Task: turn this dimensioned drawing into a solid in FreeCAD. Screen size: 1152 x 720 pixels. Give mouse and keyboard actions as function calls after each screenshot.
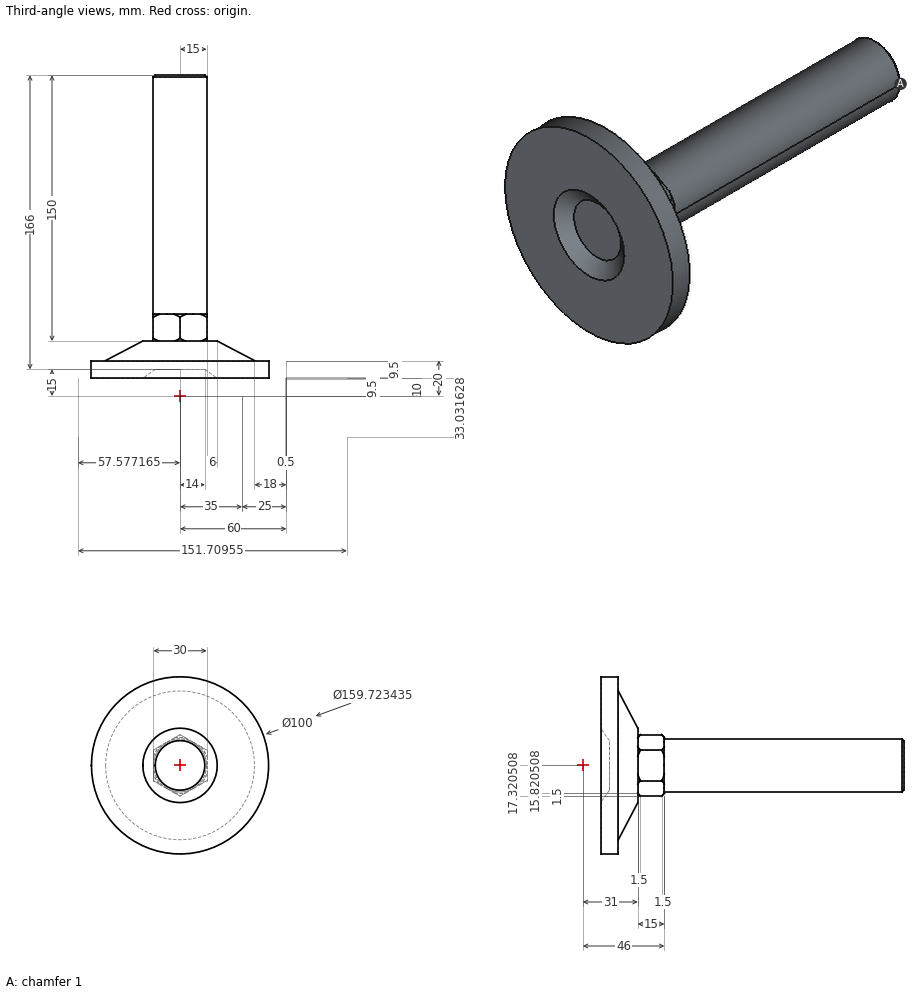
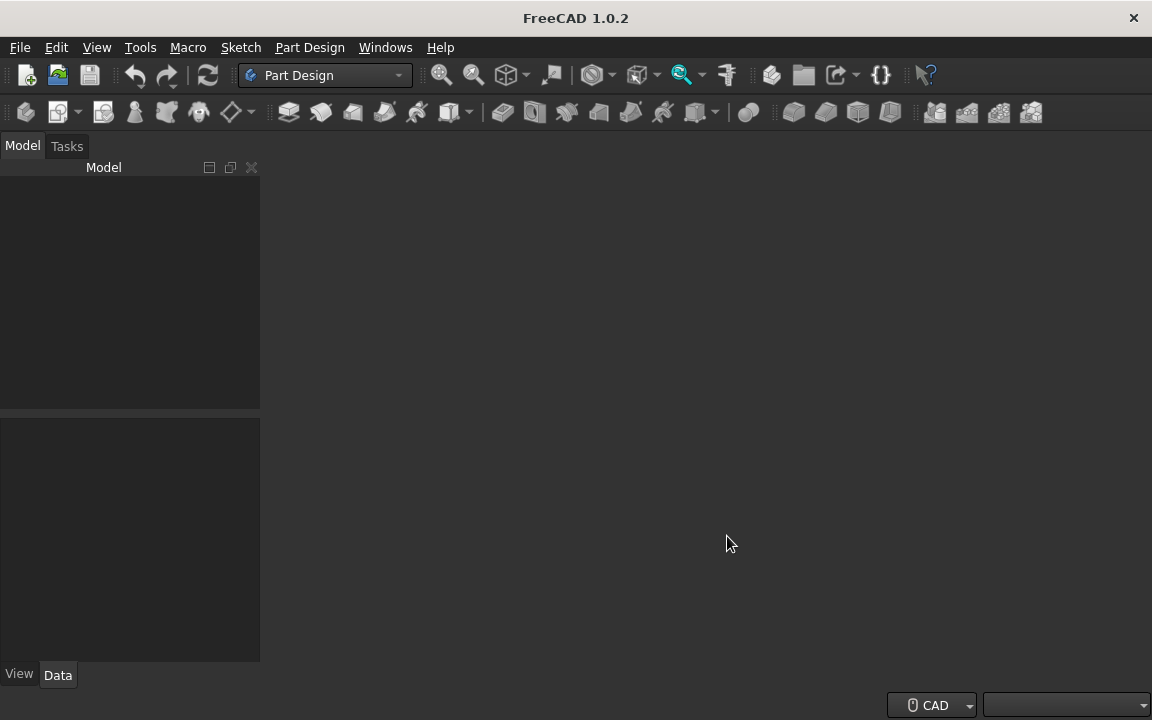
click(26, 76)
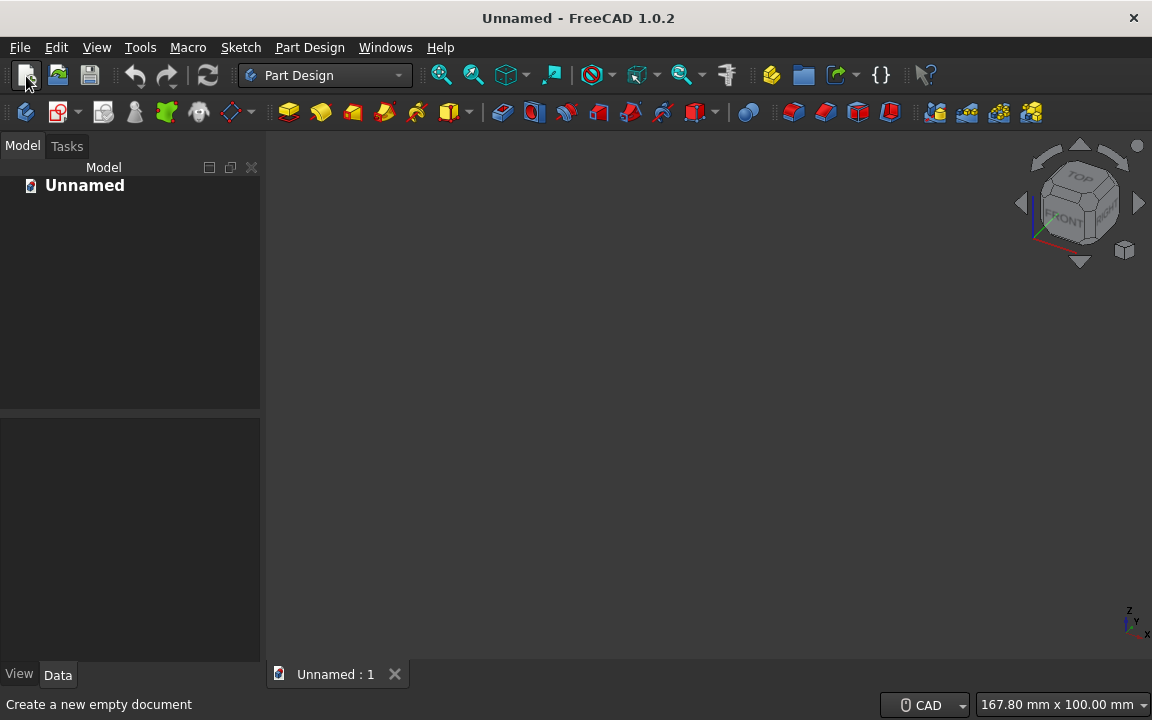
click(58, 112)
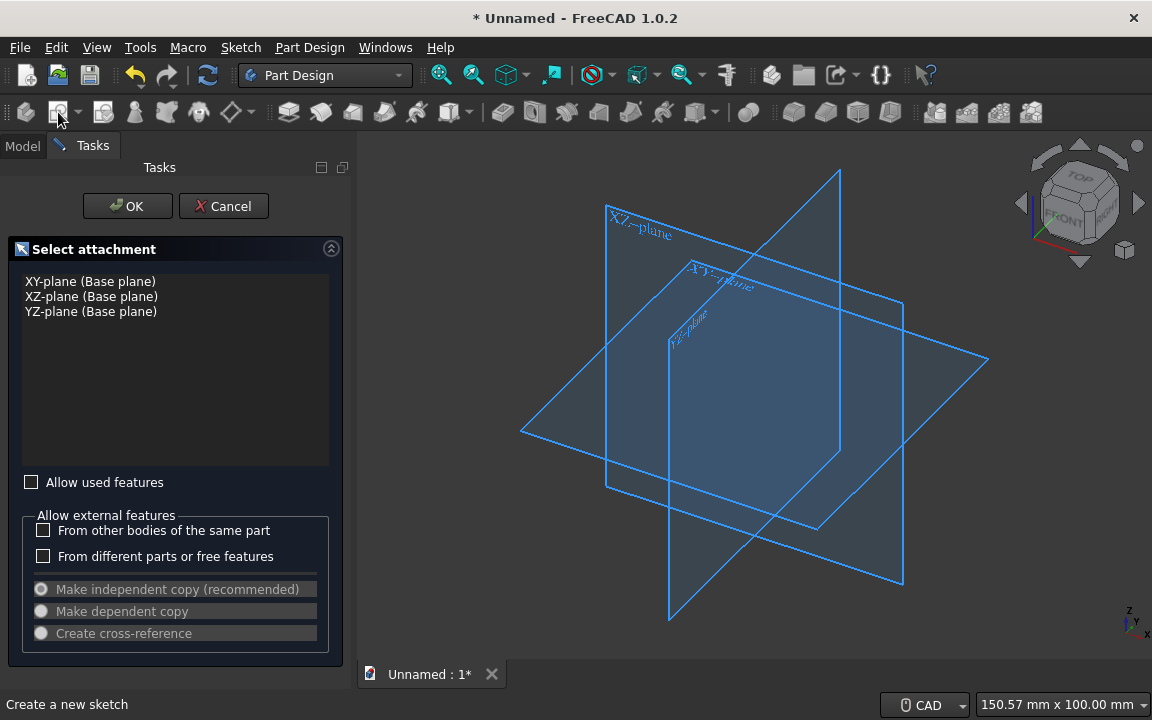
click(82, 282)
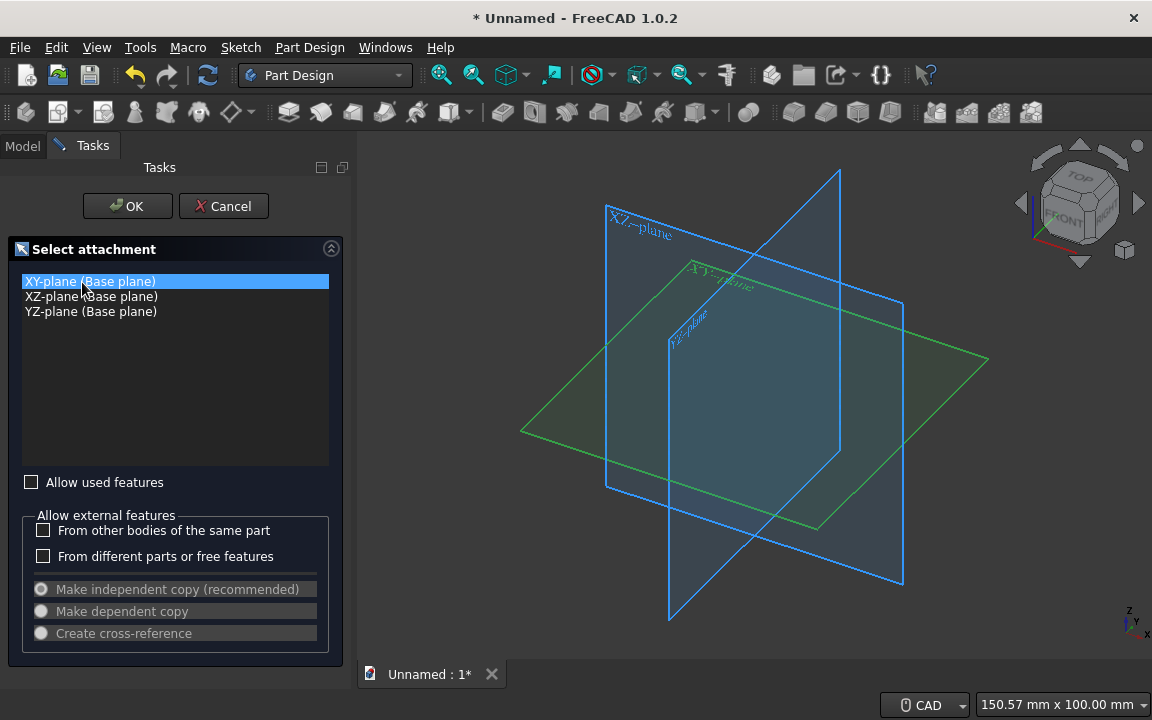
click(128, 206)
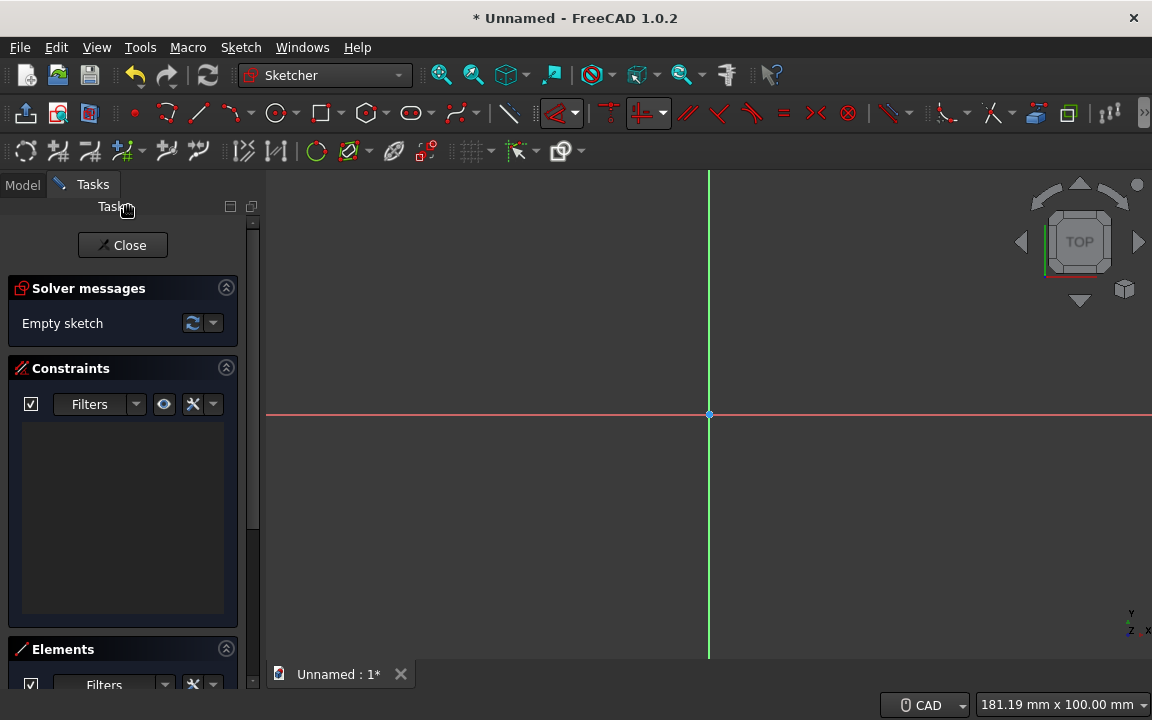
scroll(515, 631, down, 5)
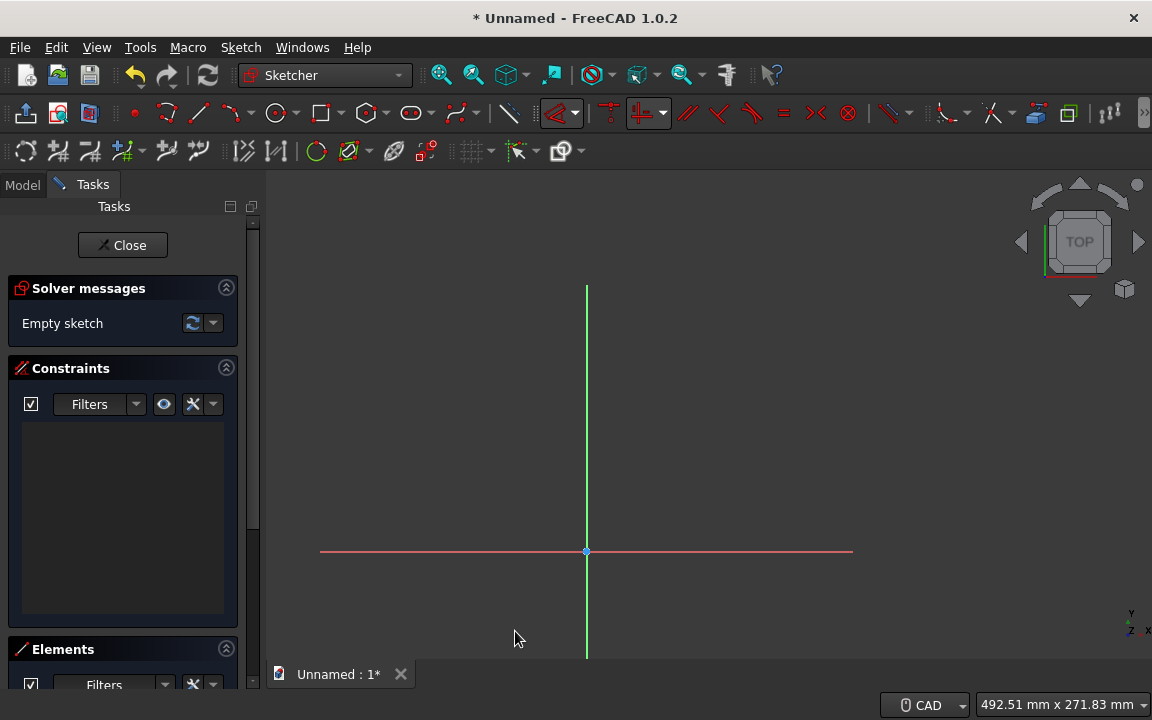
click(168, 114)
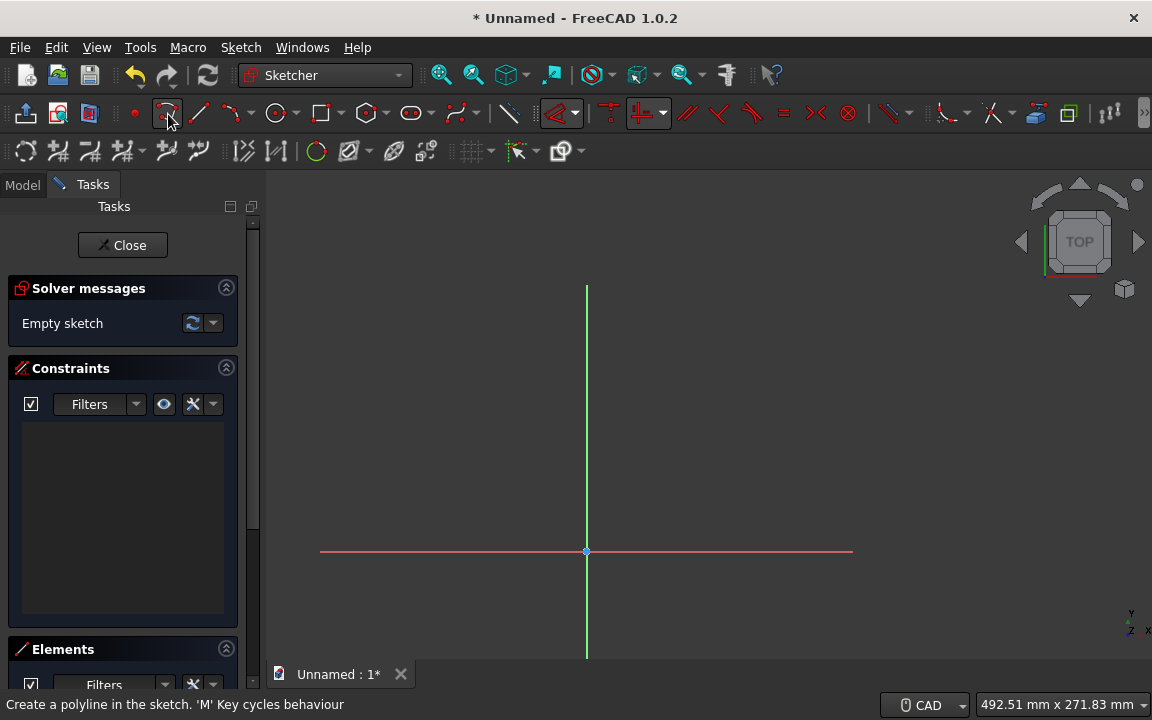
click(587, 525)
click(612, 525)
click(650, 552)
click(694, 543)
click(694, 535)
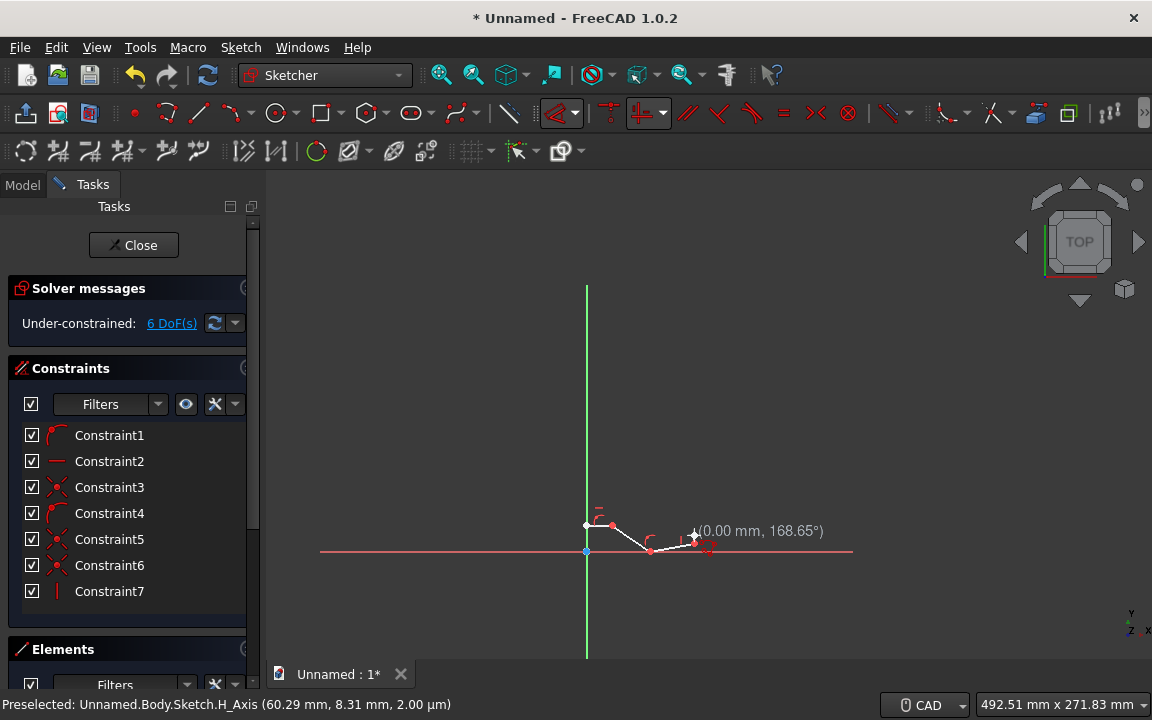
scroll(694, 534, up, 13)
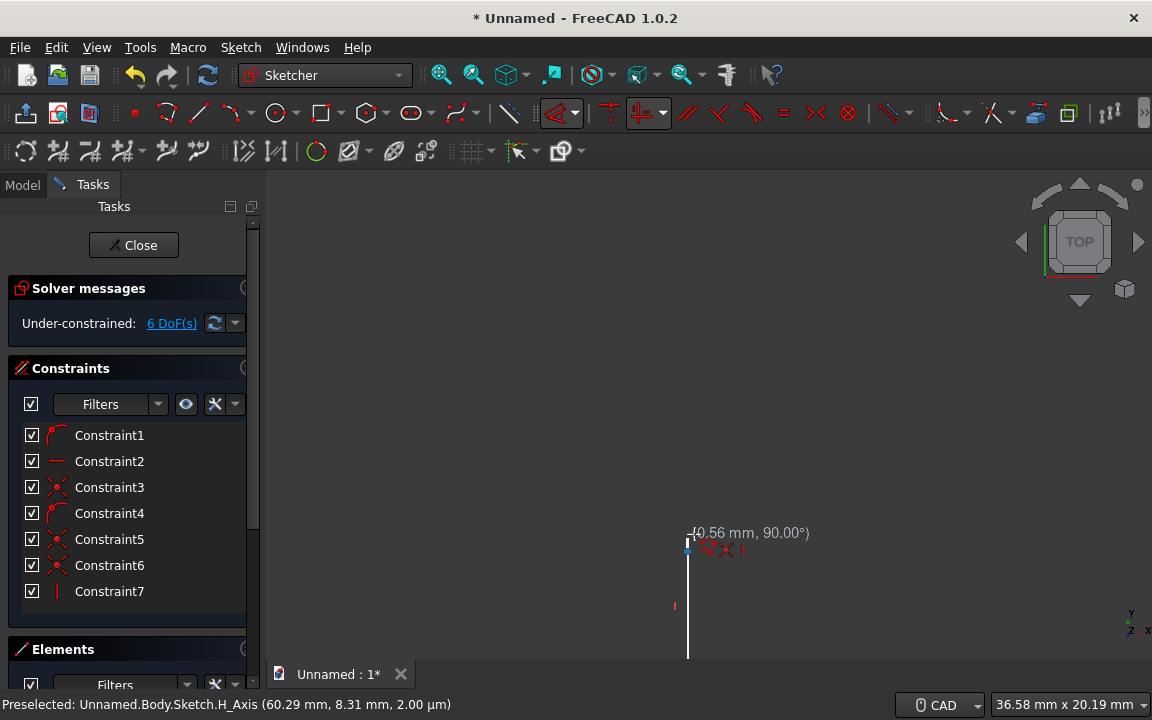
click(682, 524)
click(694, 512)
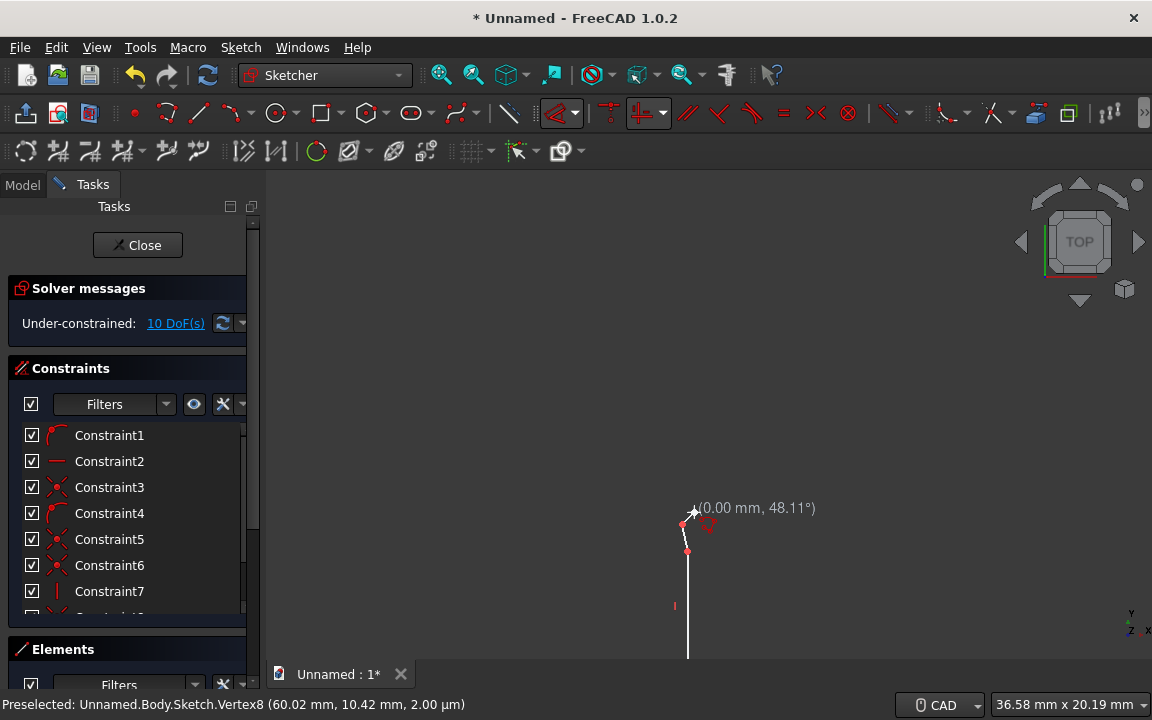
scroll(694, 562, down, 13)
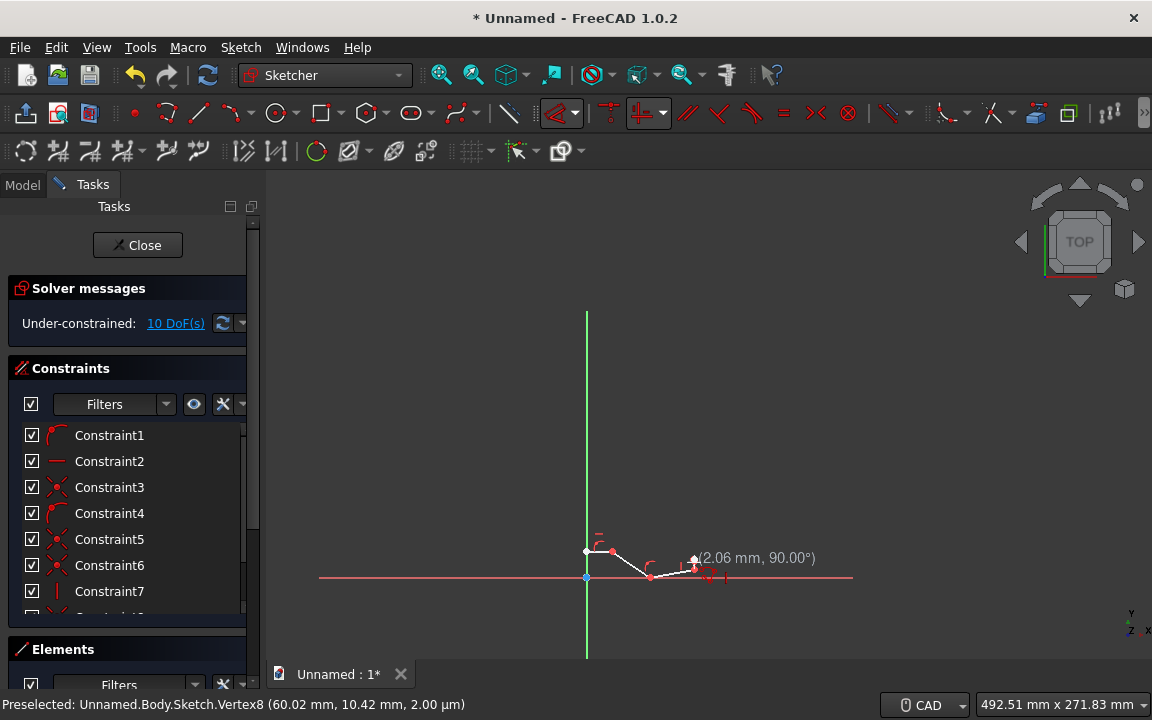
click(694, 542)
click(662, 542)
click(624, 522)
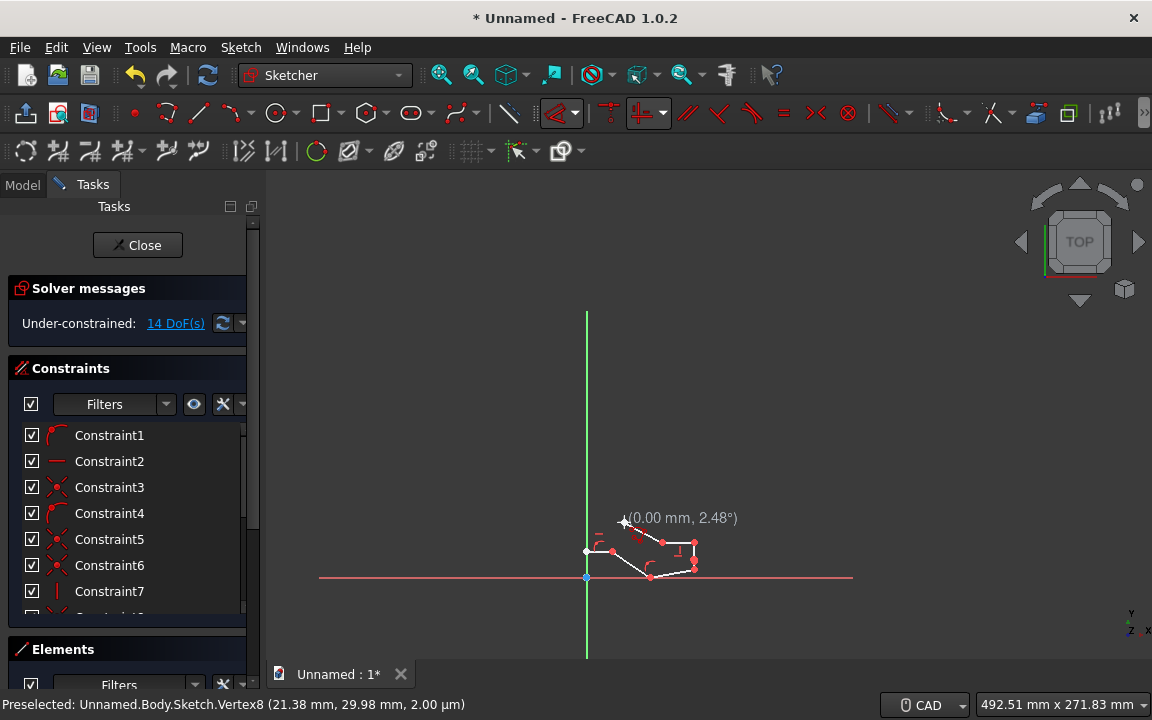
scroll(614, 522, up, 2)